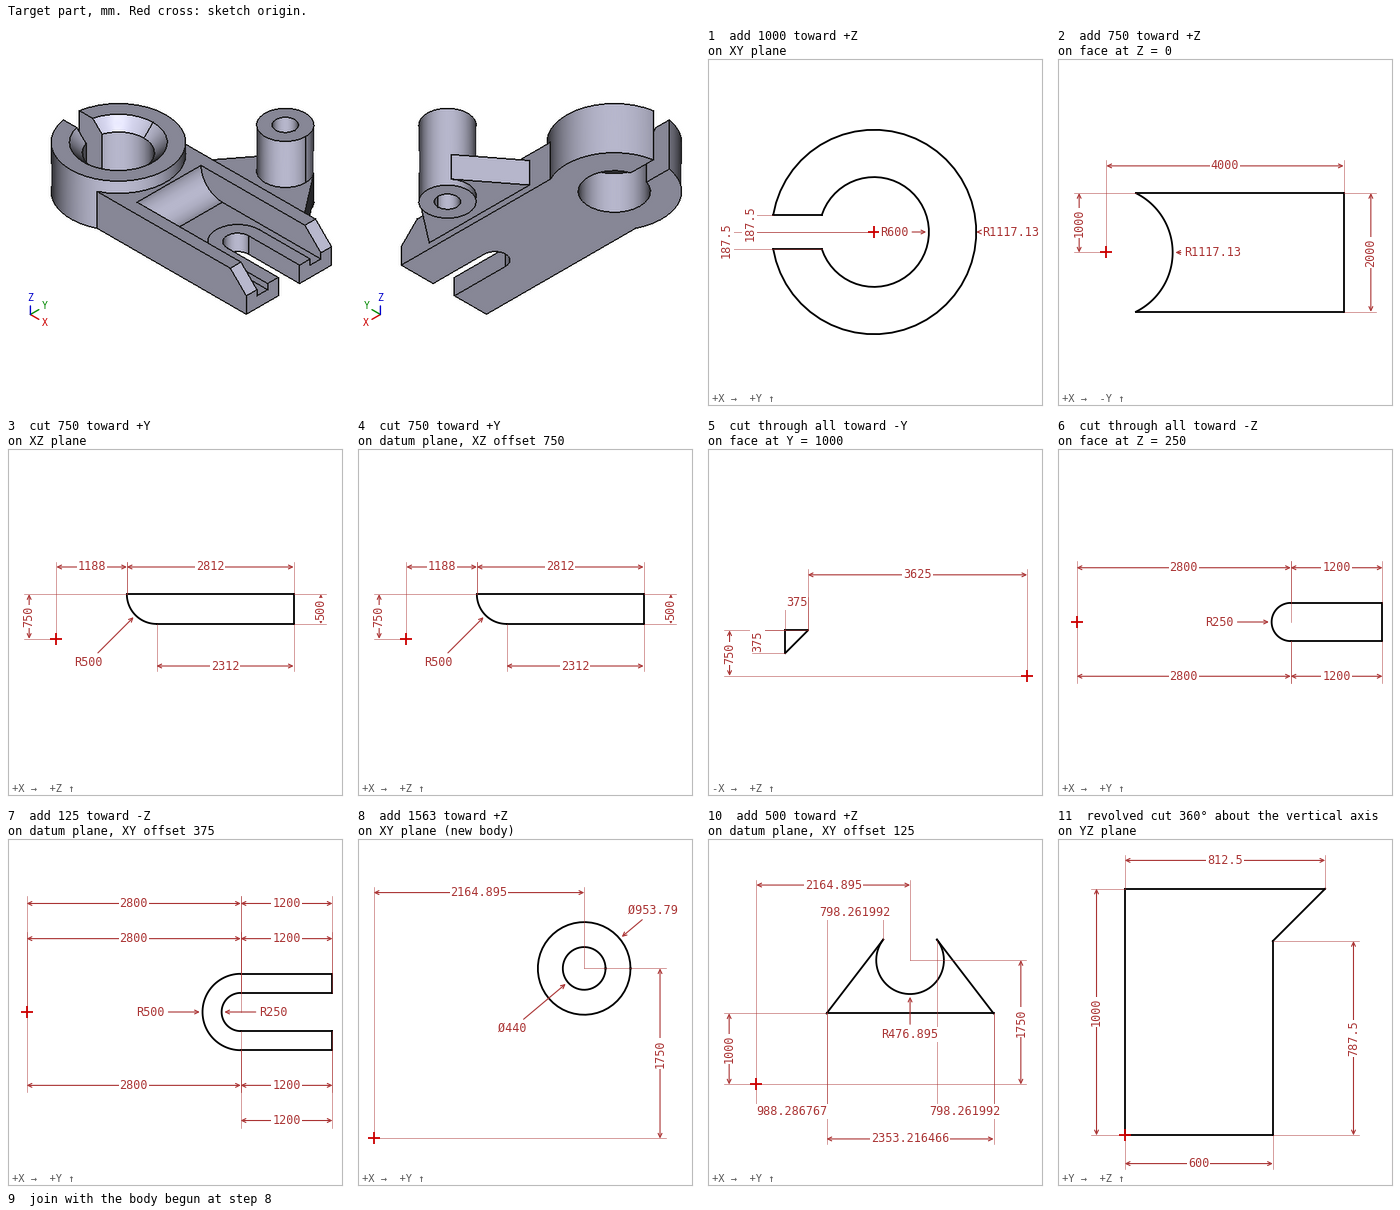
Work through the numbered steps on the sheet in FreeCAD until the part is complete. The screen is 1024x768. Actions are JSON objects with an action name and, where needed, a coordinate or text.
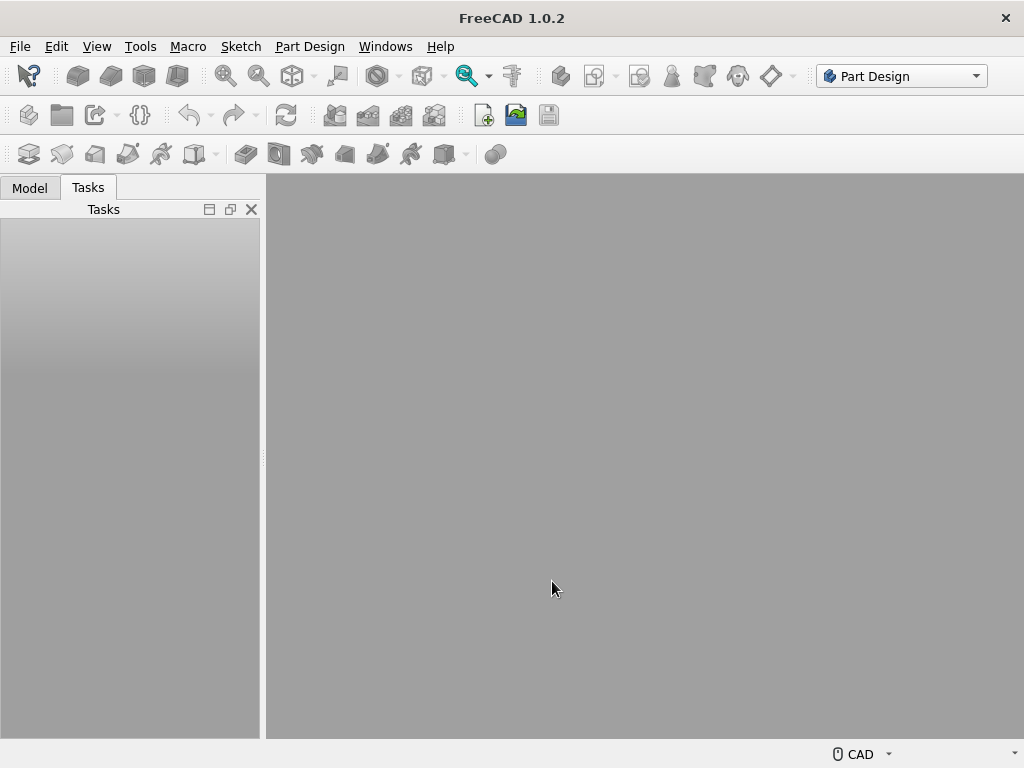
{"action": "key", "text": "ctrl+n"}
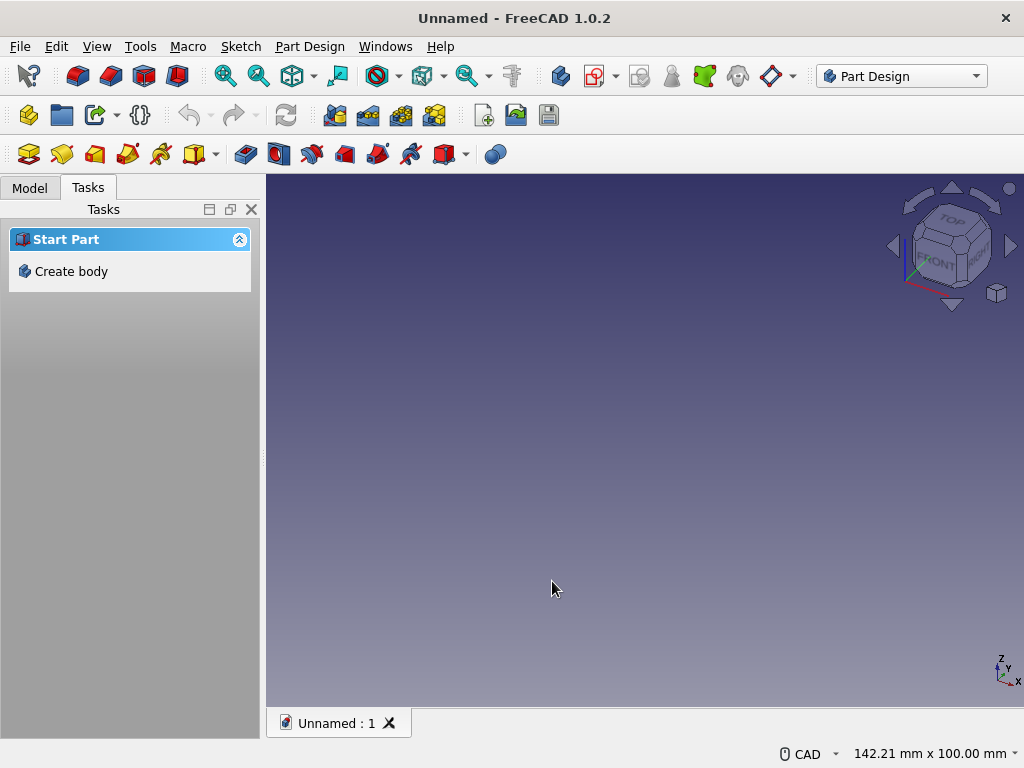
{"action": "left_click", "coordinate": [594, 76]}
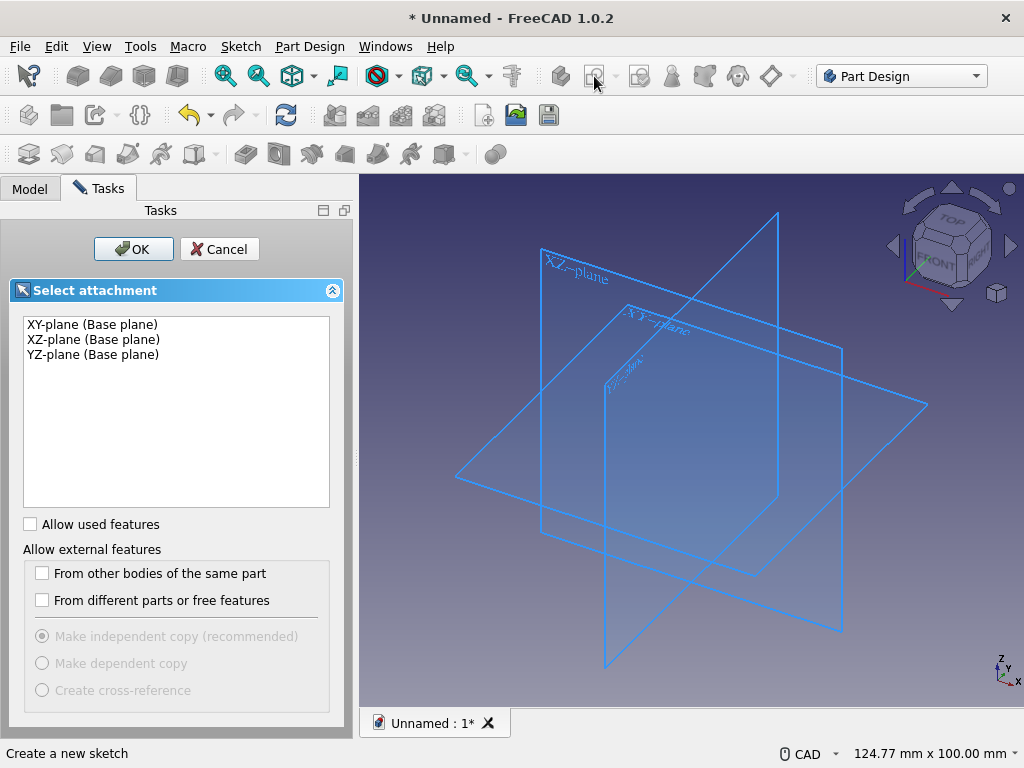
{"action": "left_click", "coordinate": [84, 324]}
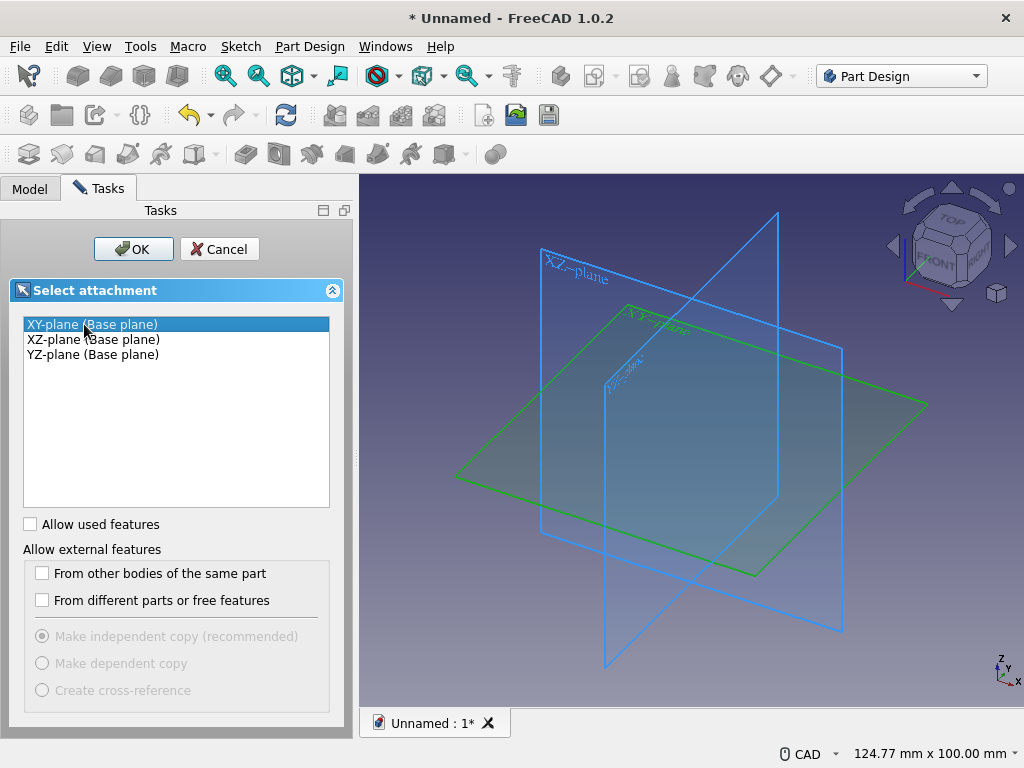
{"action": "left_click", "coordinate": [134, 249]}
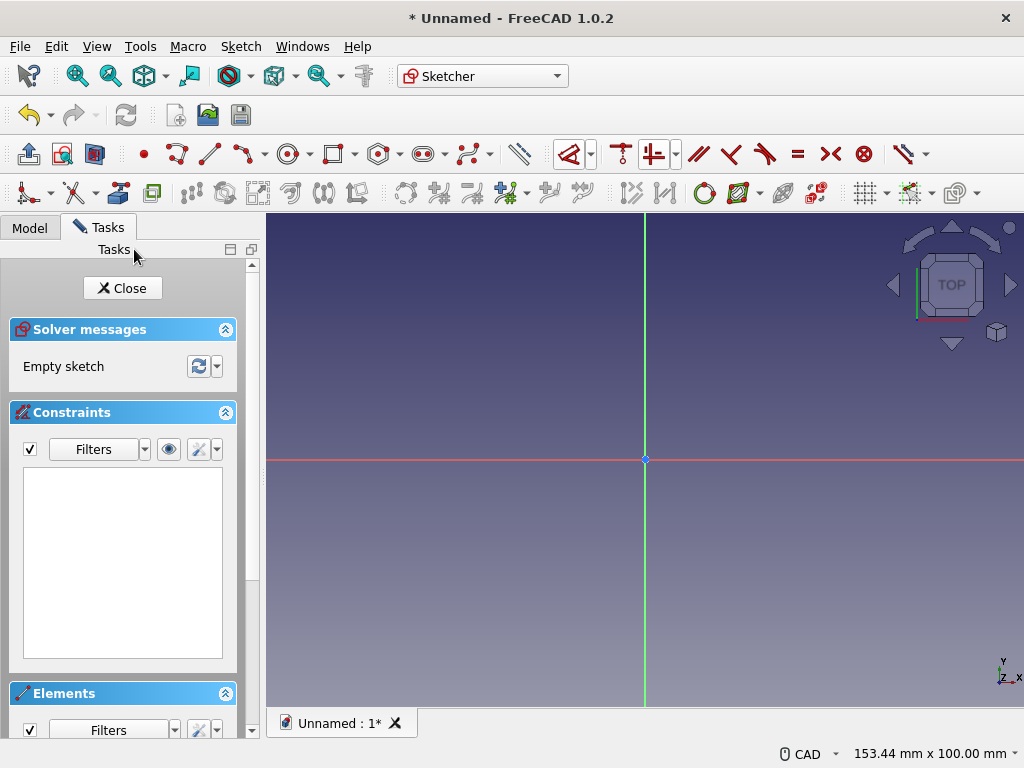
{"action": "scroll", "coordinate": [572, 460], "scroll_direction": "down", "scroll_amount": 16}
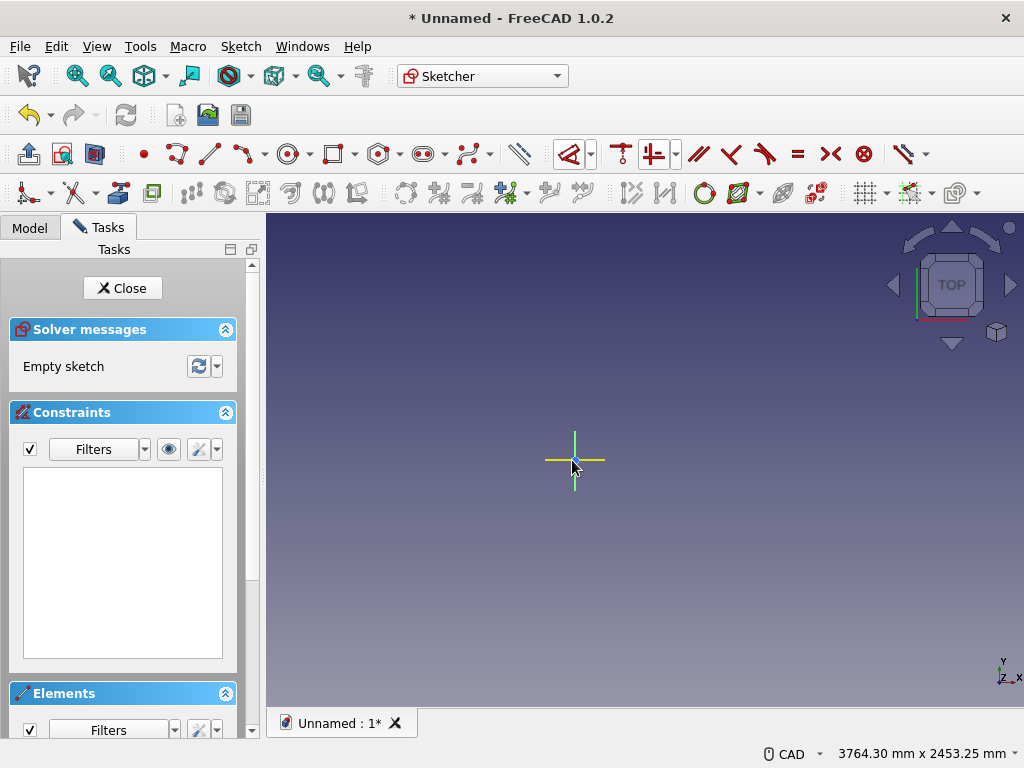
{"action": "key", "text": "g l"}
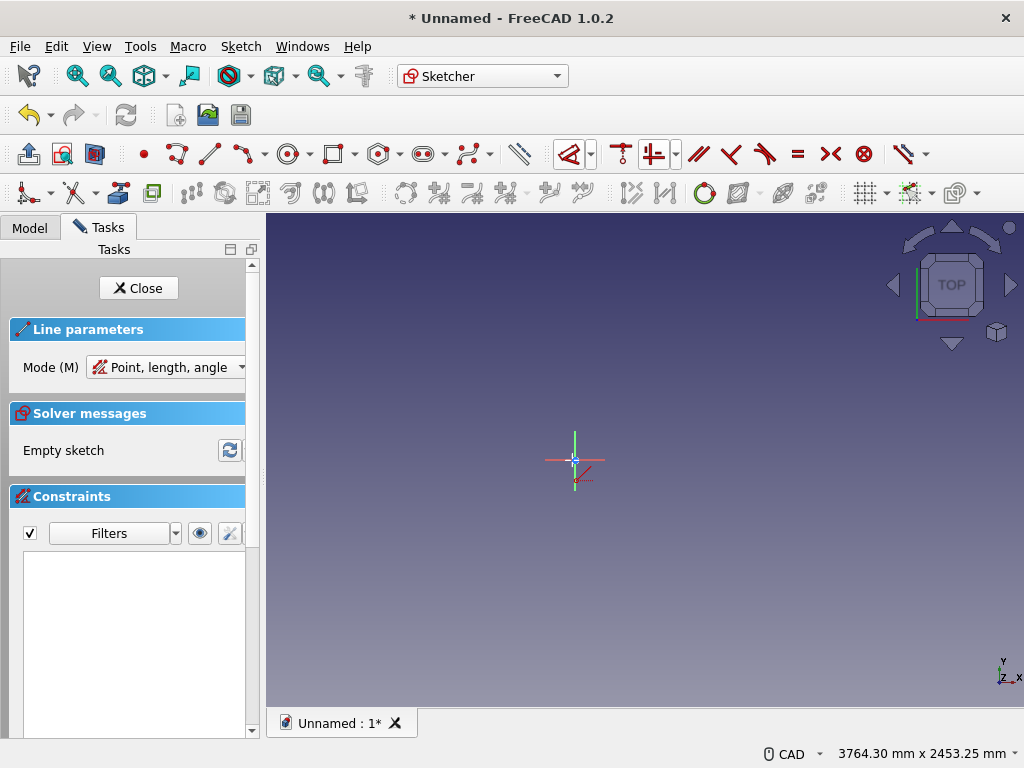
{"action": "left_click", "coordinate": [354, 423]}
{"action": "left_click", "coordinate": [461, 423]}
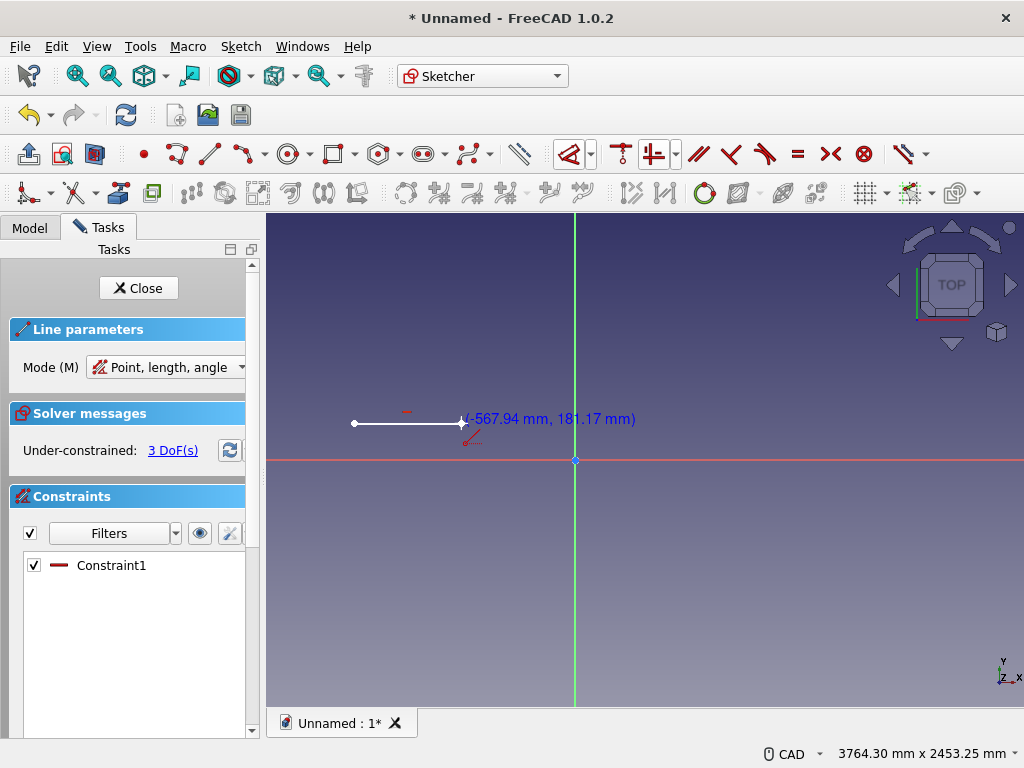
{"action": "left_click", "coordinate": [461, 498]}
{"action": "left_click", "coordinate": [354, 498]}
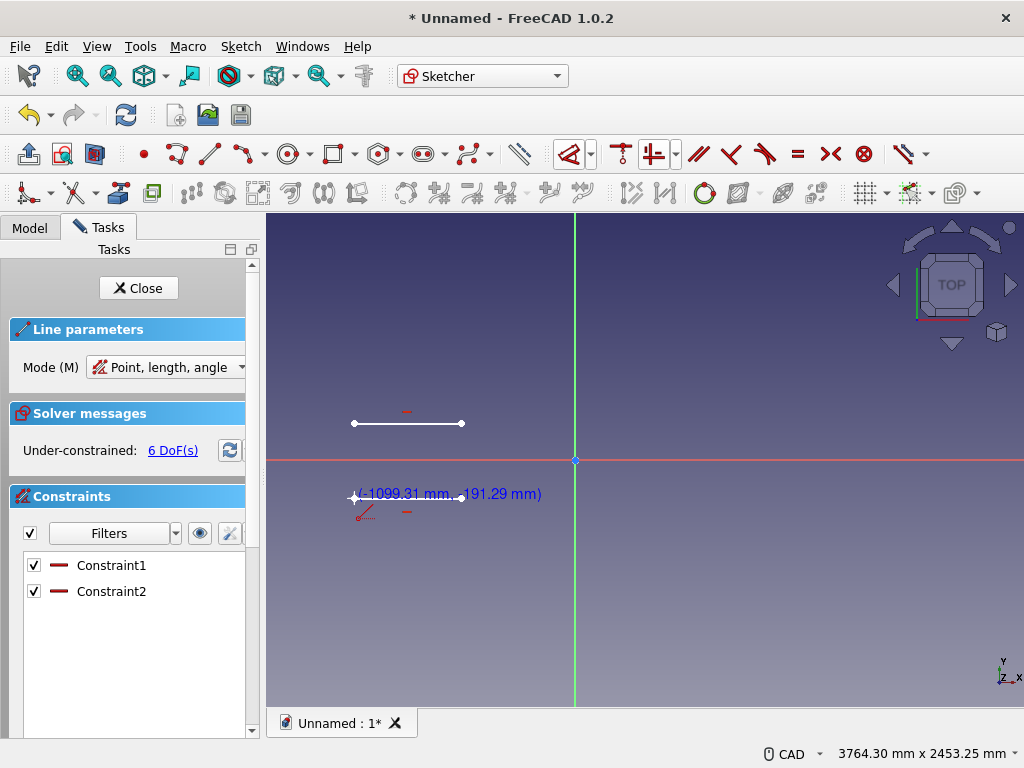
{"action": "left_click", "coordinate": [242, 154]}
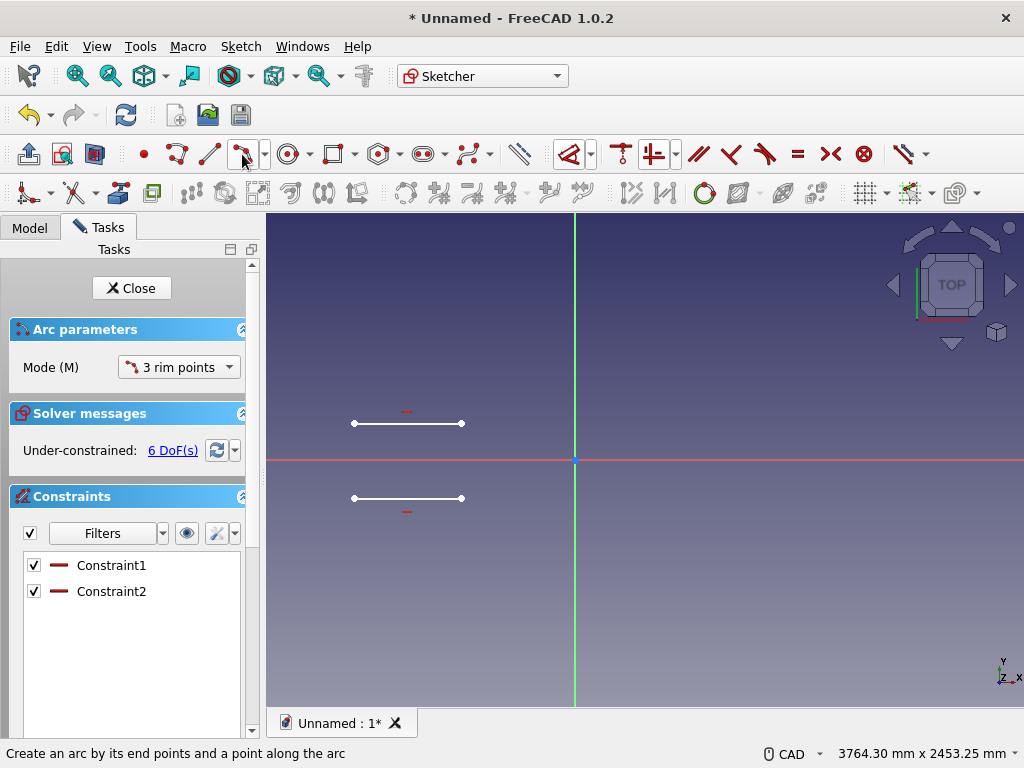
{"action": "left_click", "coordinate": [461, 424]}
{"action": "left_click", "coordinate": [461, 499]}
{"action": "left_click", "coordinate": [677, 525]}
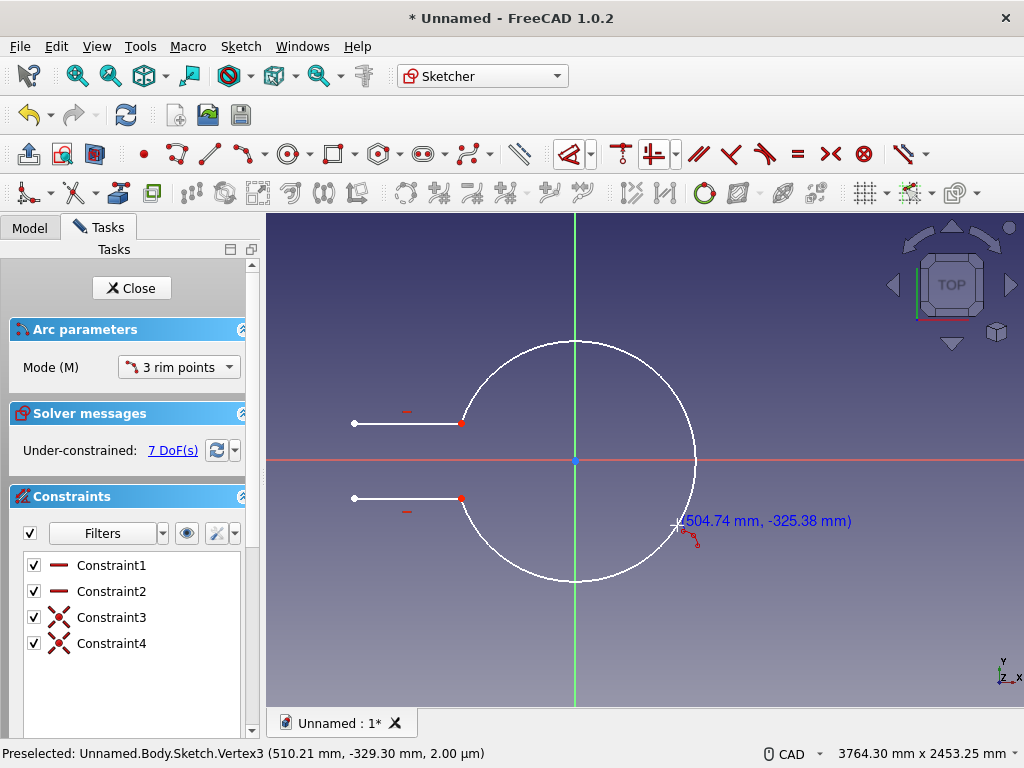
{"action": "left_click", "coordinate": [354, 499]}
{"action": "left_click", "coordinate": [354, 424]}
{"action": "left_click", "coordinate": [762, 586]}
{"action": "key", "text": "Escape"}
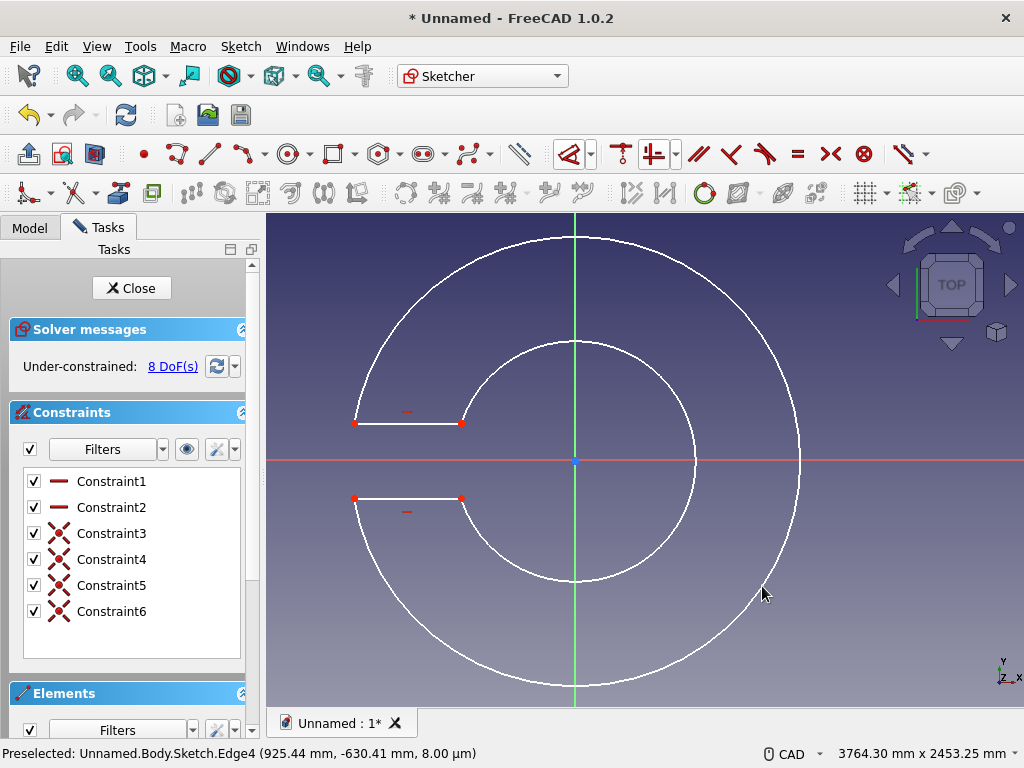
{"action": "left_click", "coordinate": [627, 570]}